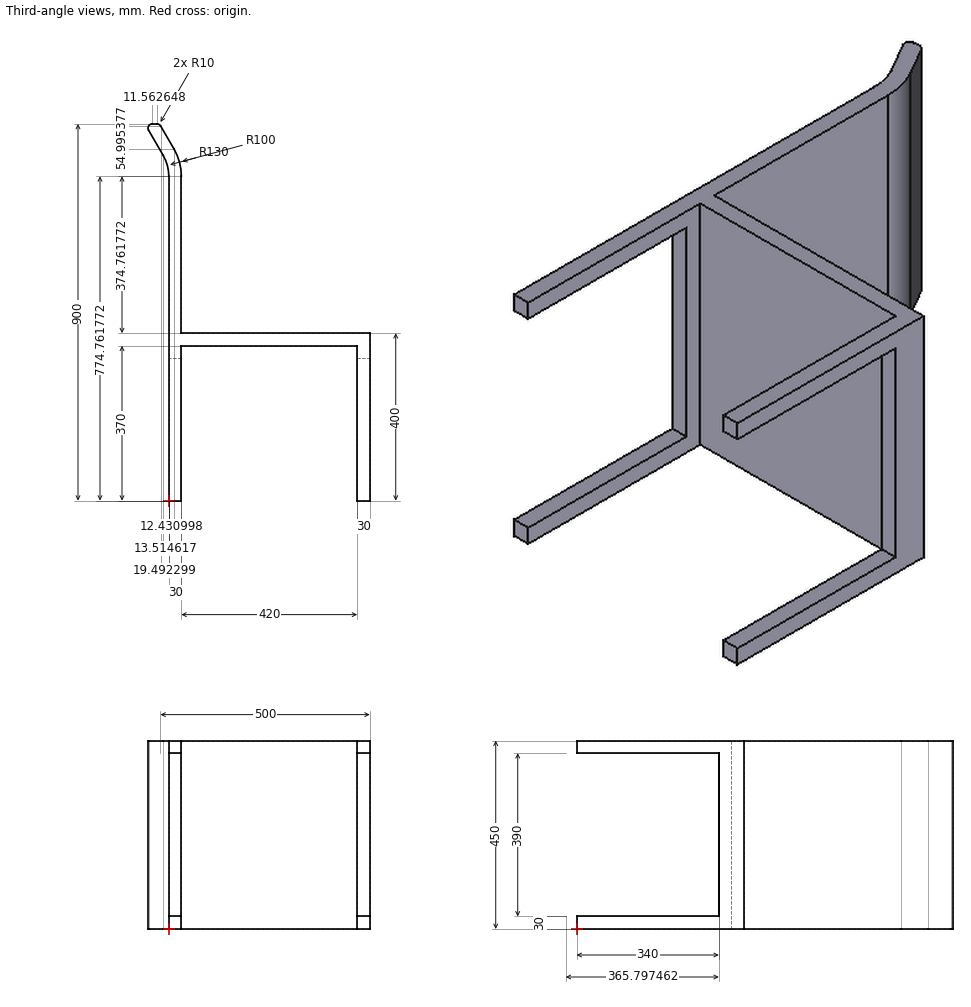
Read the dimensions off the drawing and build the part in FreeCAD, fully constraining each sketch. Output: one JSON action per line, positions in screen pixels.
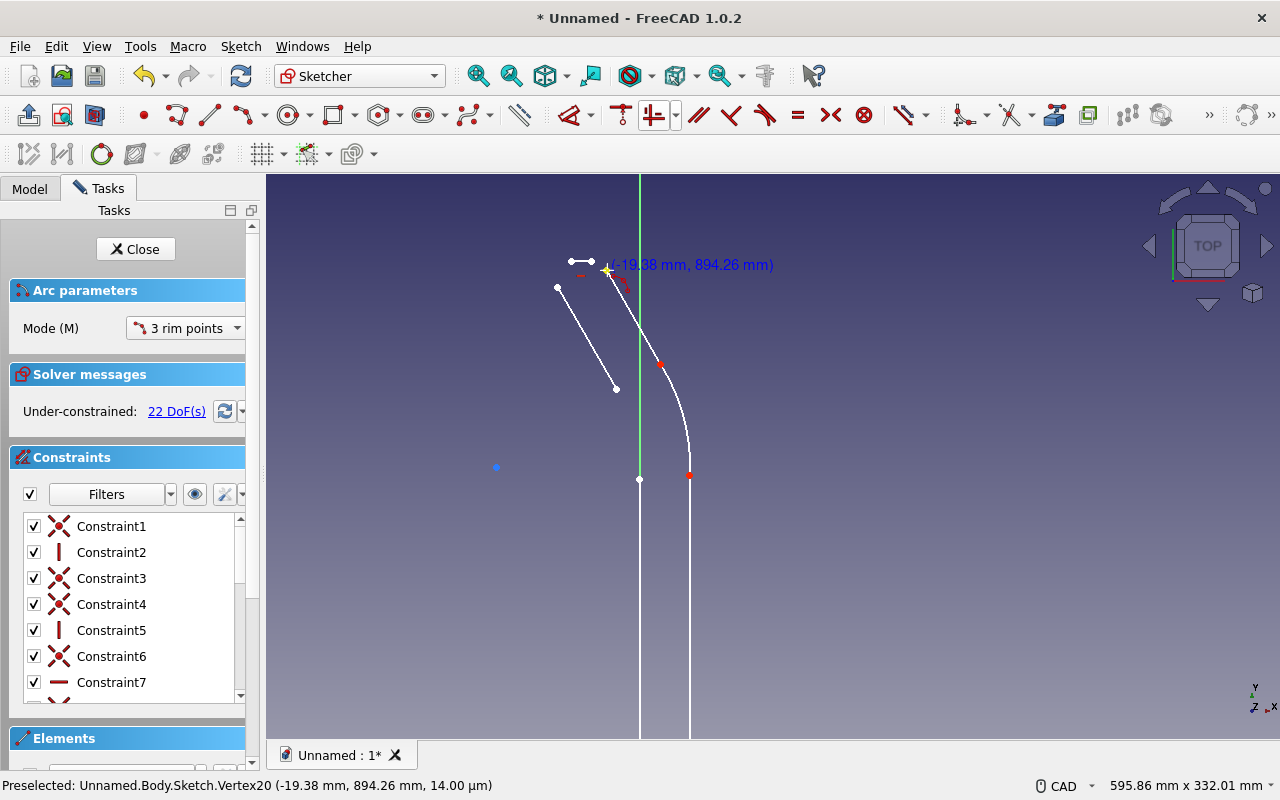
{"action": "scroll", "coordinate": [592, 260], "scroll_direction": "up", "scroll_amount": 3}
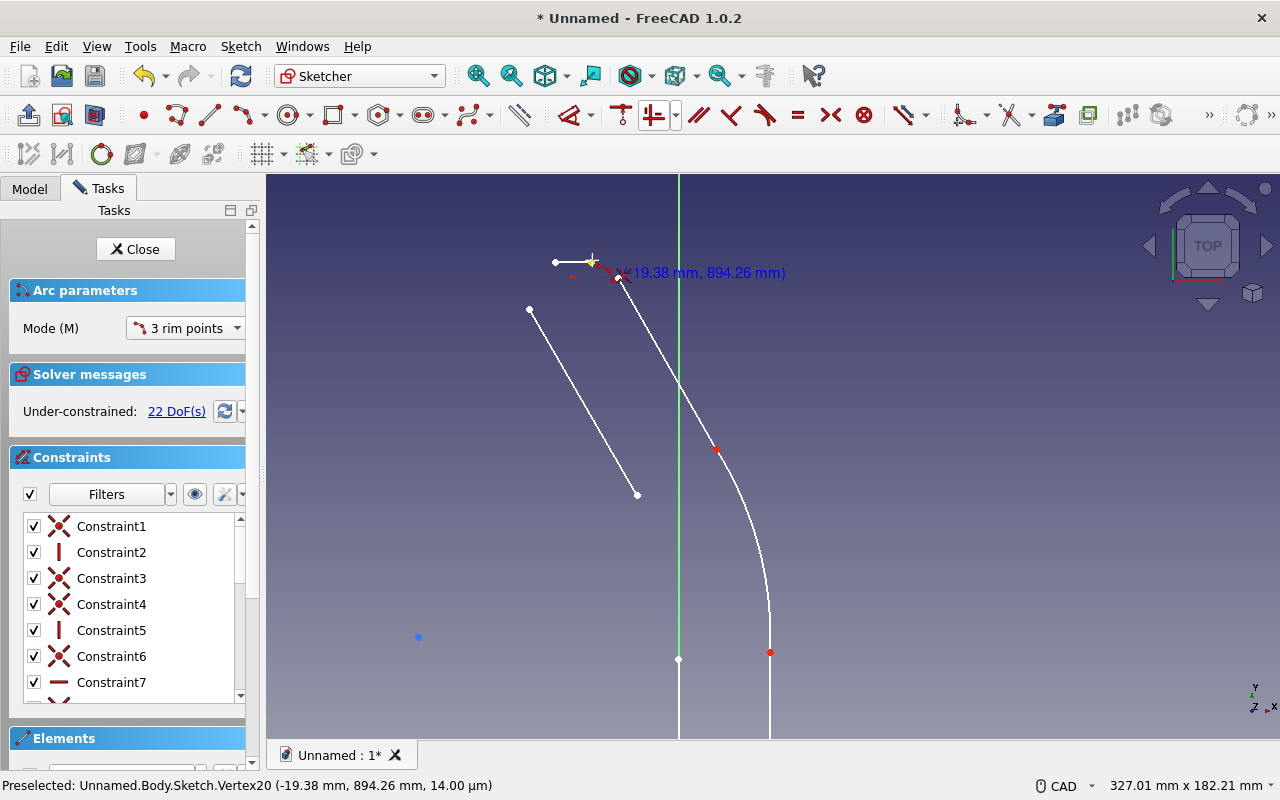
{"action": "left_click", "coordinate": [591, 262]}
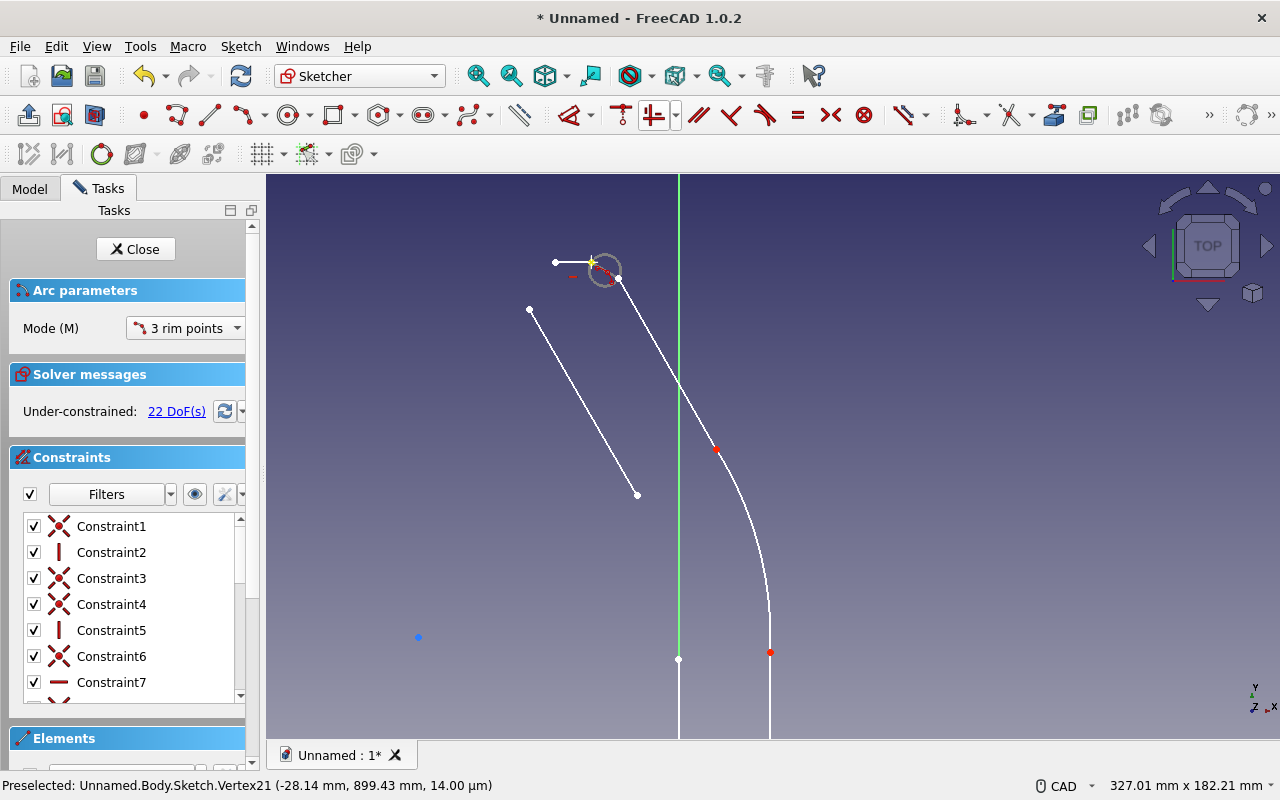
{"action": "scroll", "coordinate": [607, 265], "scroll_direction": "up", "scroll_amount": 7}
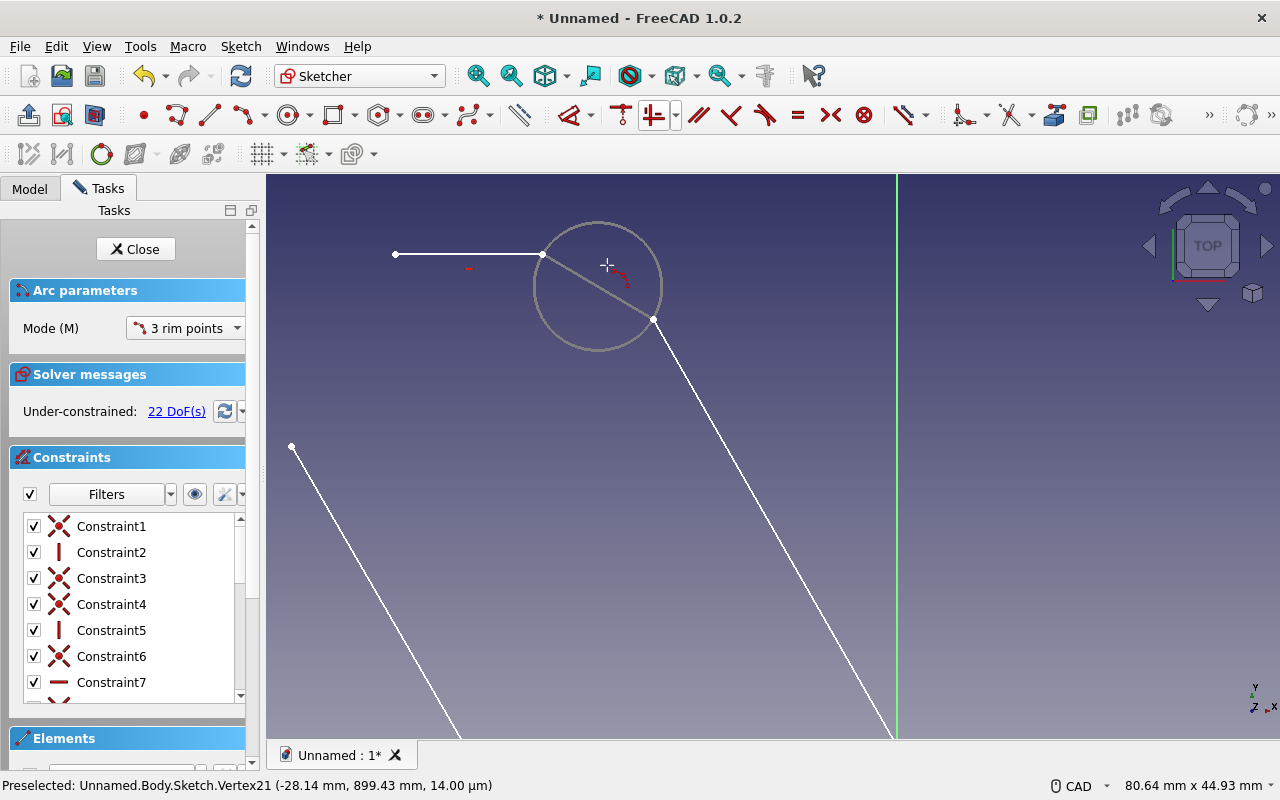
{"action": "left_click", "coordinate": [606, 264]}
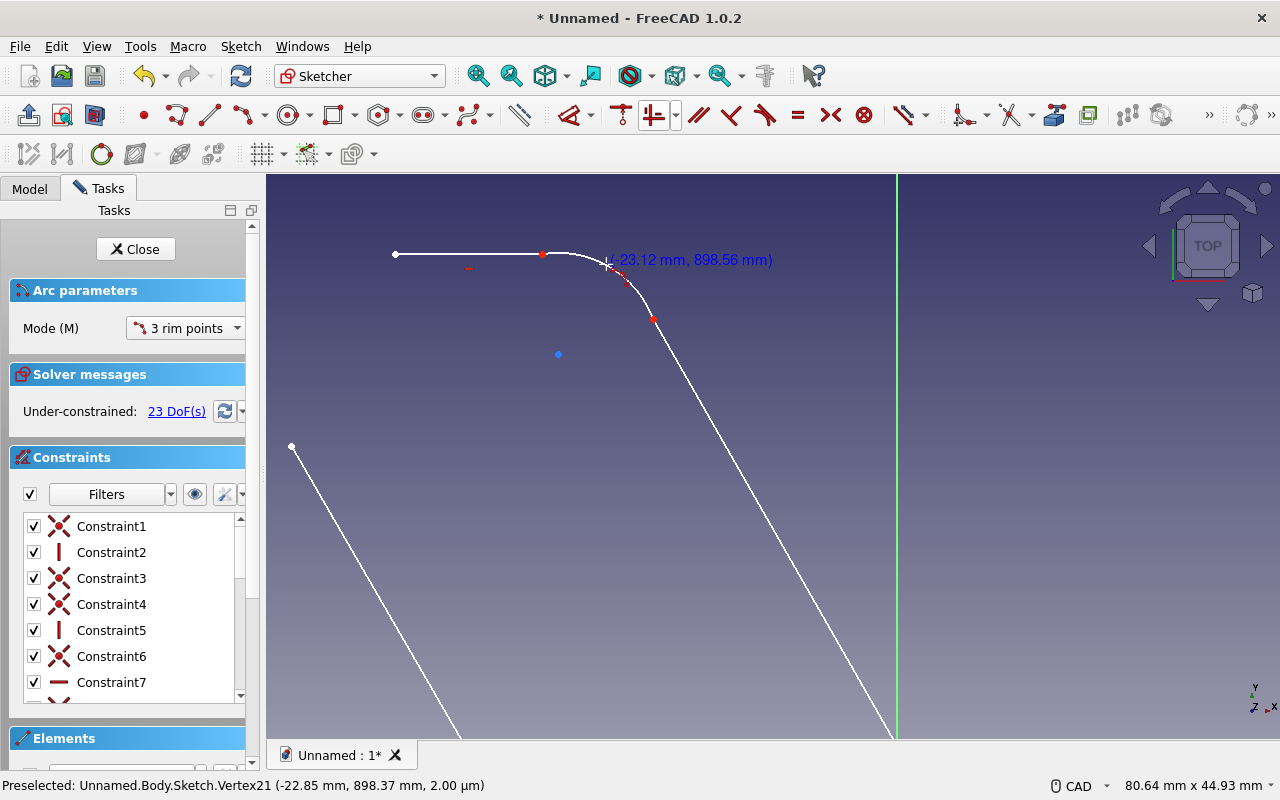
{"action": "scroll", "coordinate": [604, 268], "scroll_direction": "down", "scroll_amount": 17}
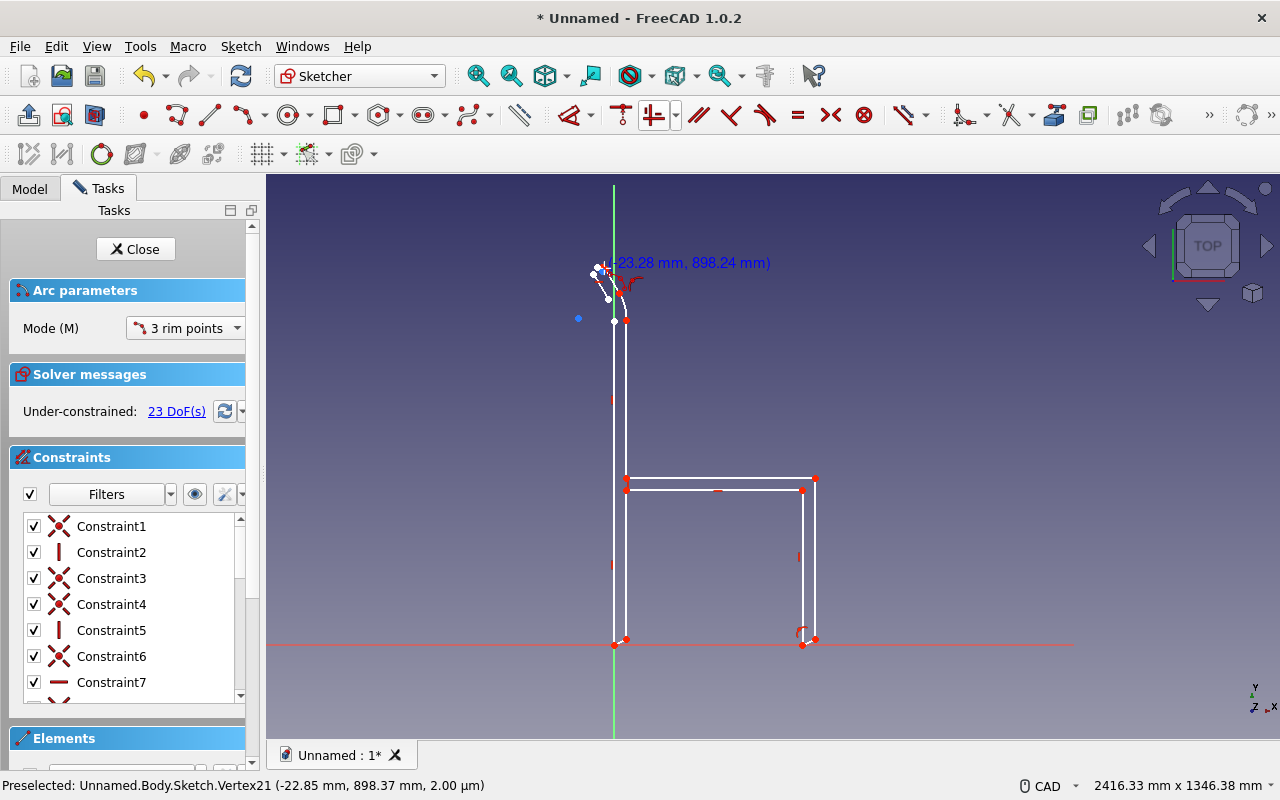
{"action": "scroll", "coordinate": [597, 267], "scroll_direction": "up", "scroll_amount": 10}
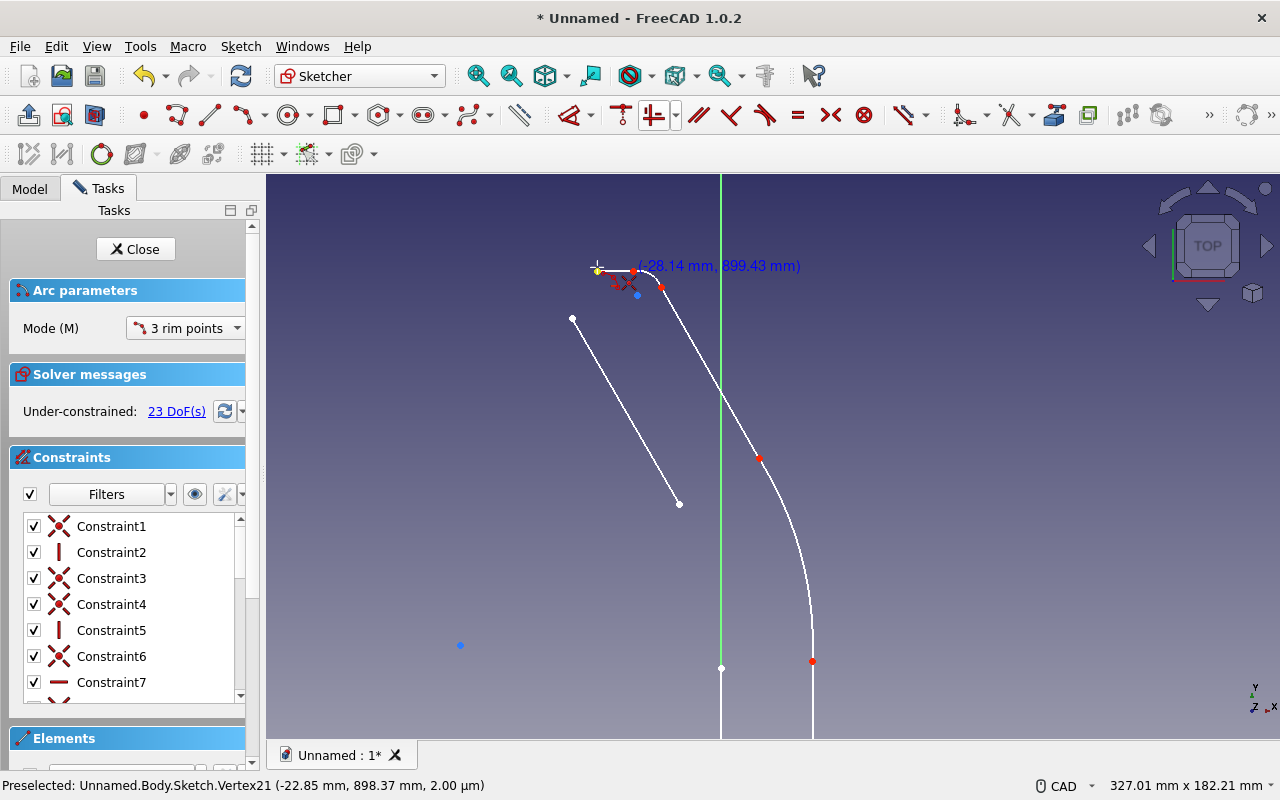
{"action": "left_click", "coordinate": [598, 271]}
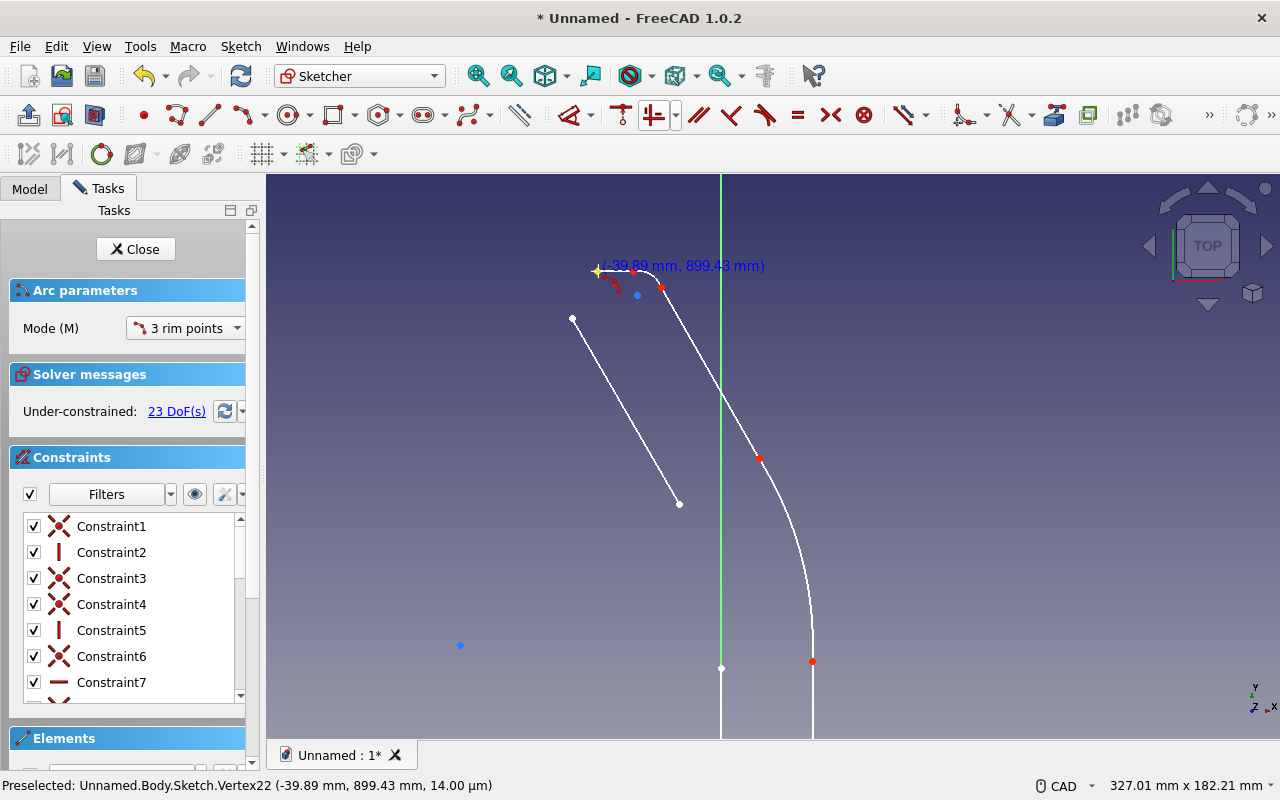
{"action": "scroll", "coordinate": [597, 267], "scroll_direction": "down", "scroll_amount": 10}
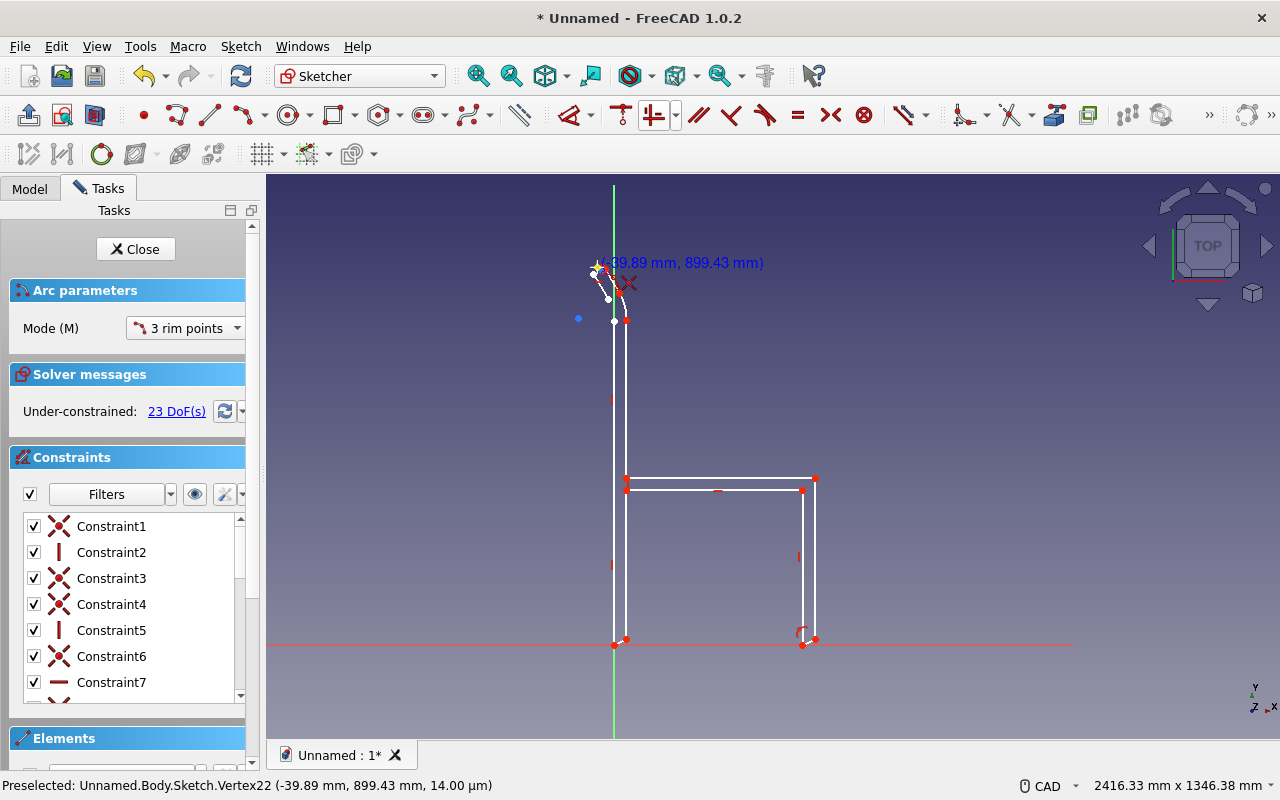
{"action": "scroll", "coordinate": [594, 274], "scroll_direction": "up", "scroll_amount": 4}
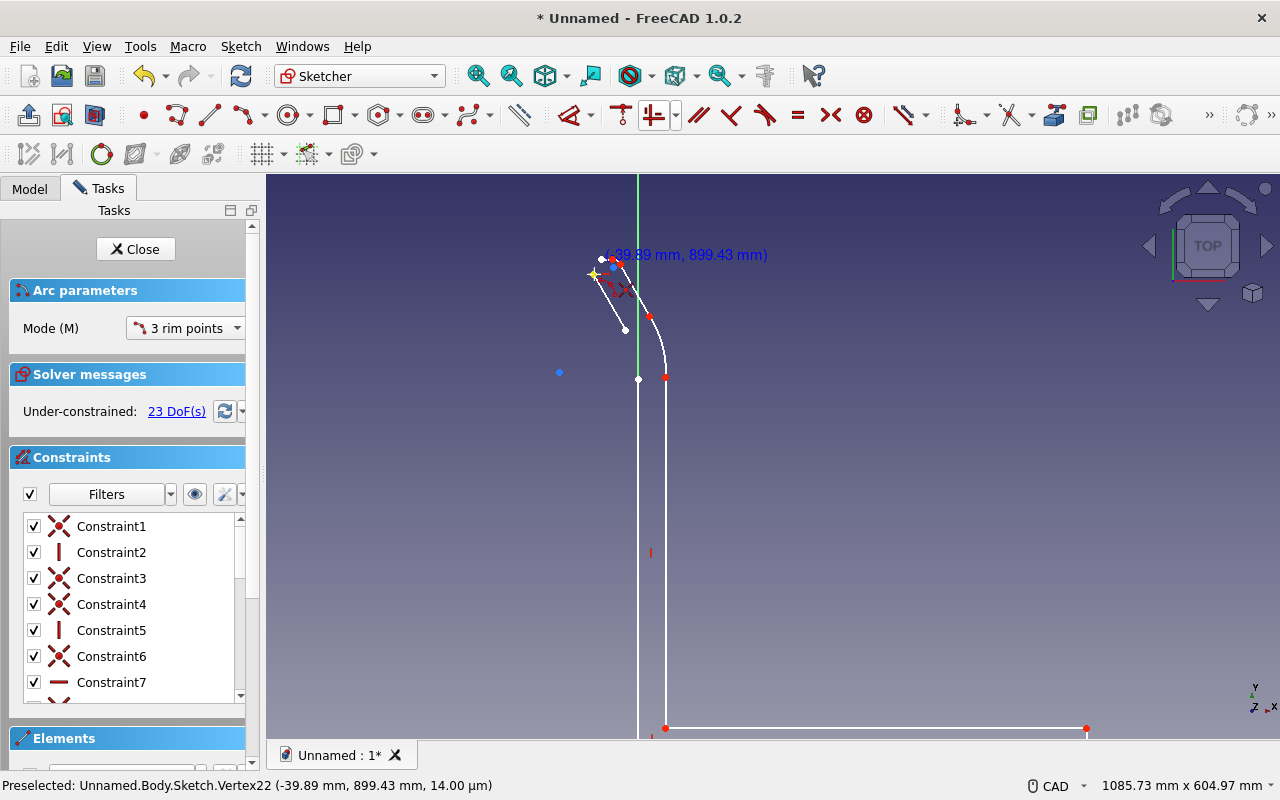
{"action": "left_click", "coordinate": [593, 274]}